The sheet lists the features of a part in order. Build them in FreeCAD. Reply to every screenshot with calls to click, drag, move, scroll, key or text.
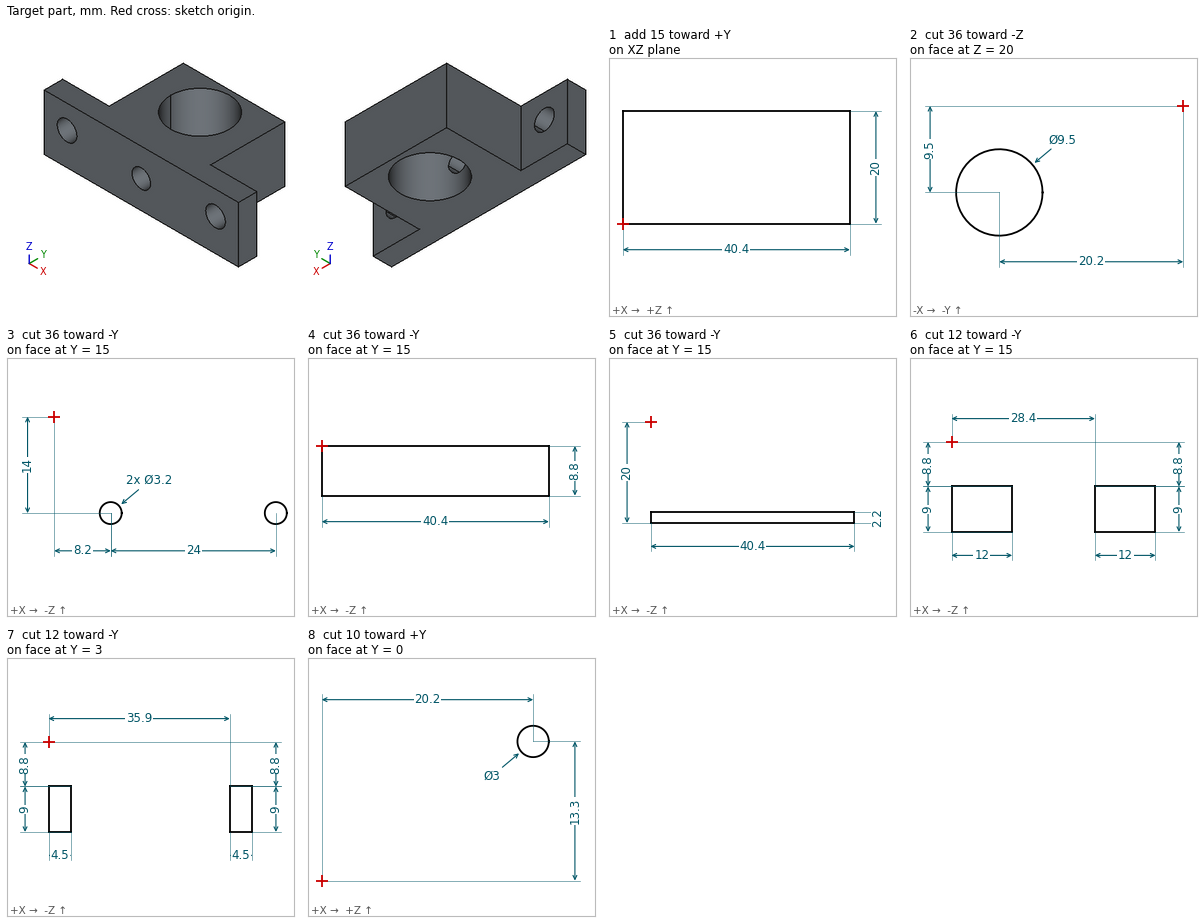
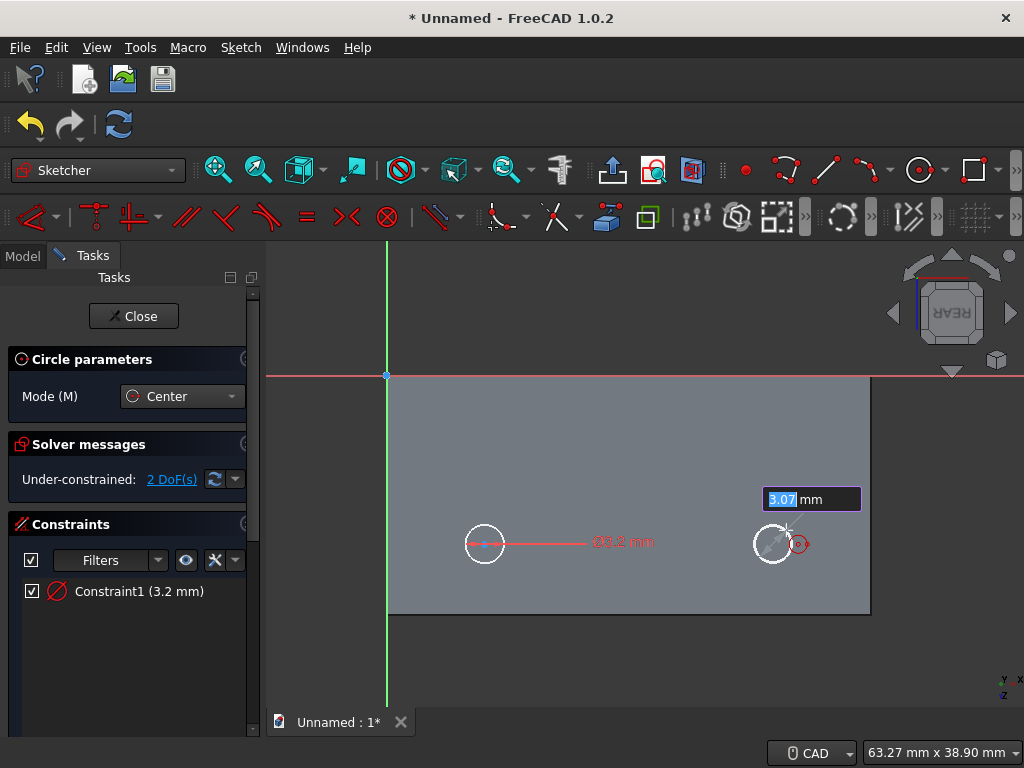
text(3.2)
key(Return)
key(Escape)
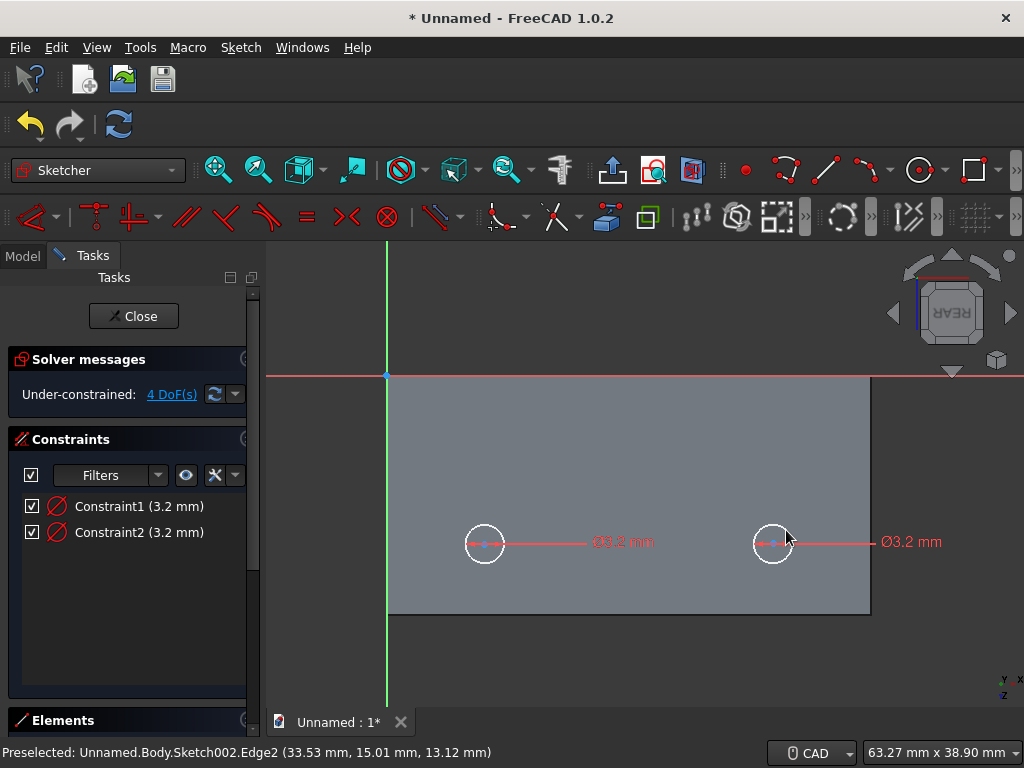
click(485, 544)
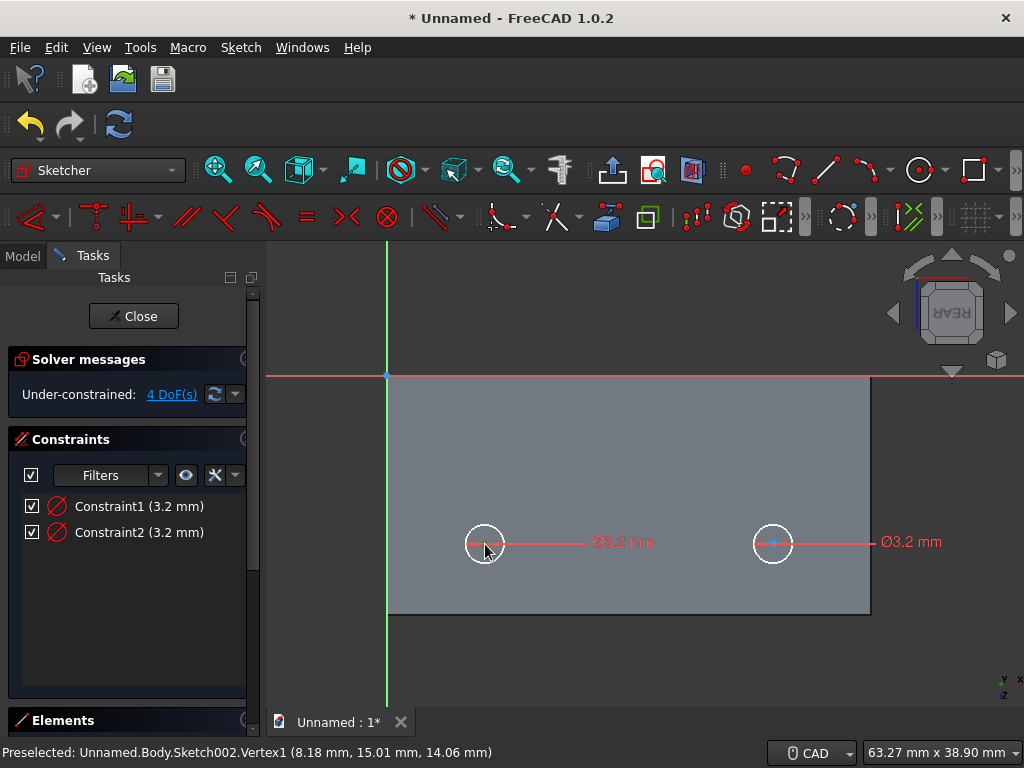
click(773, 544)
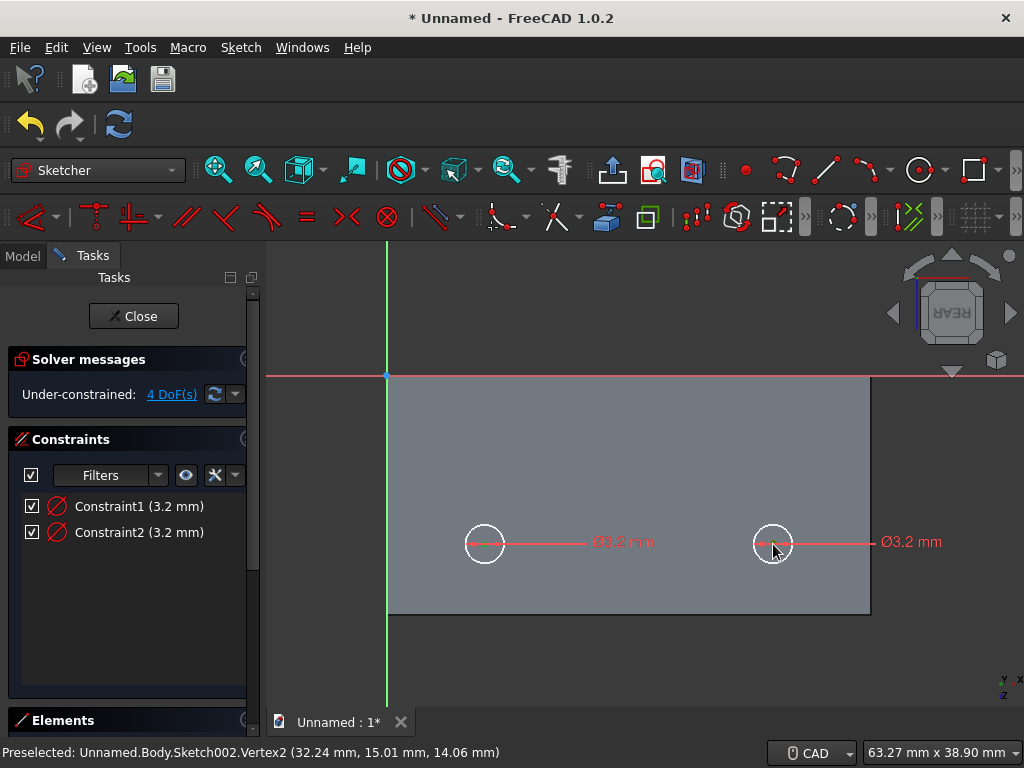
key(h)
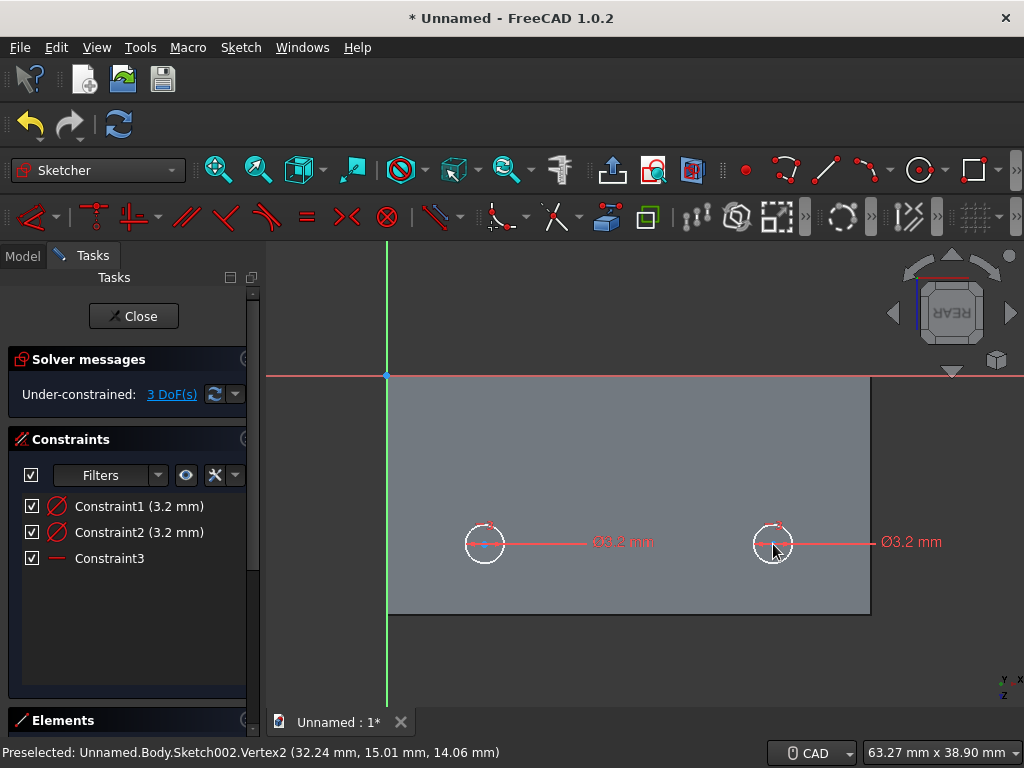
click(485, 544)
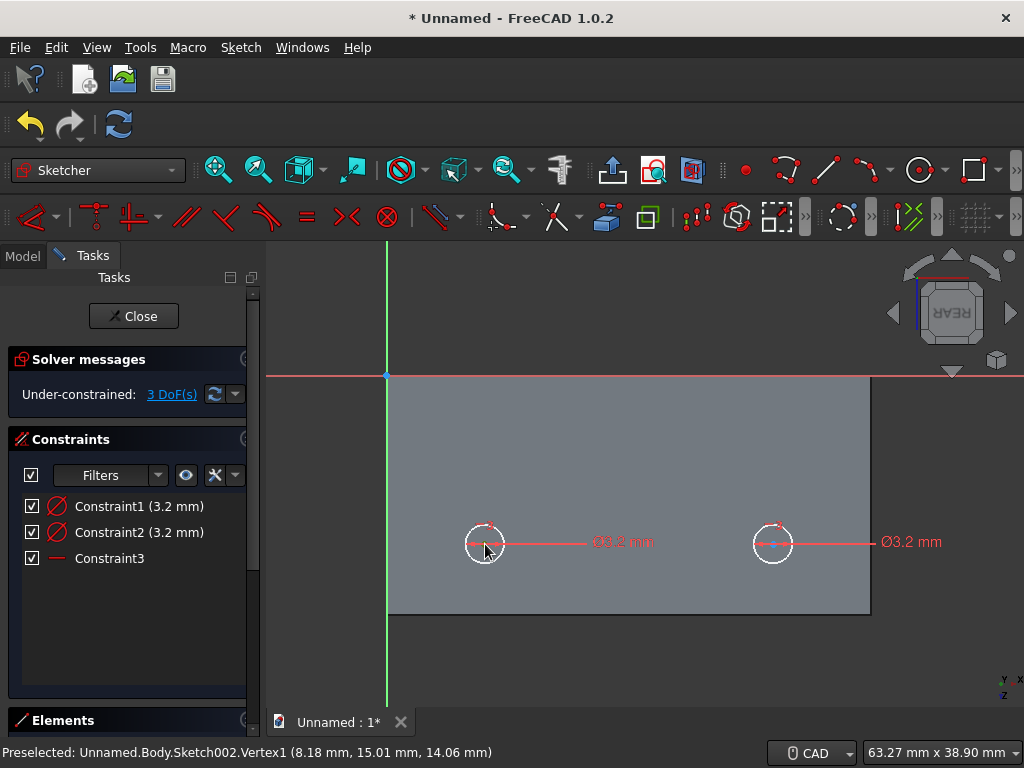
key(i)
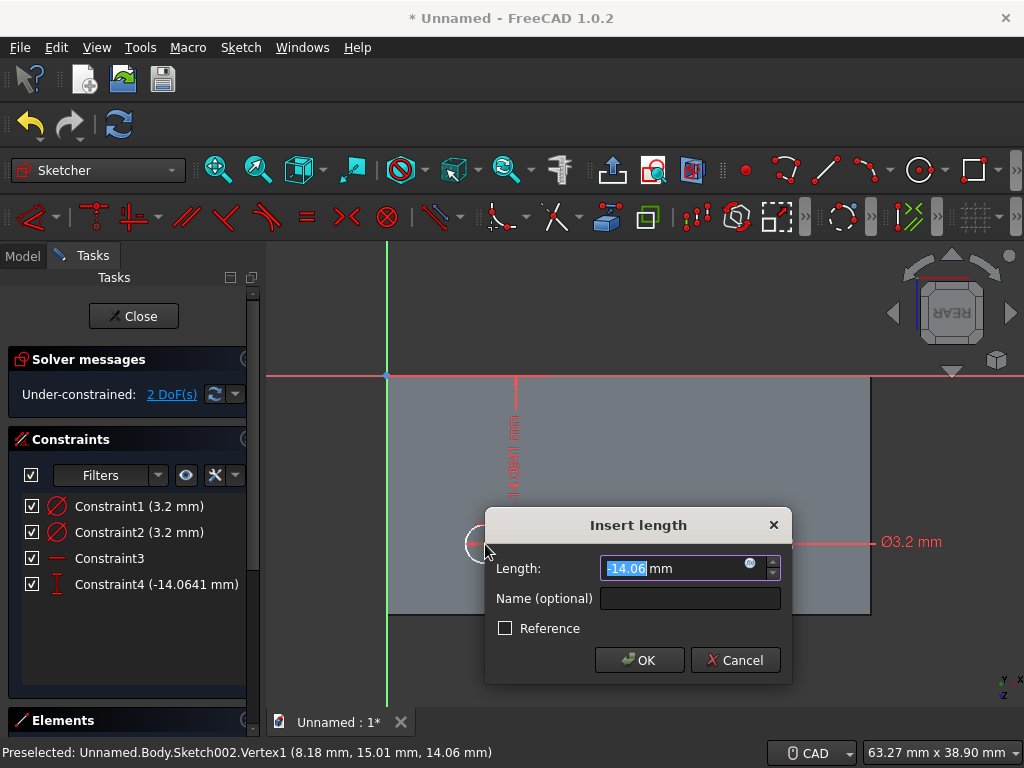
text(-14)
key(Return)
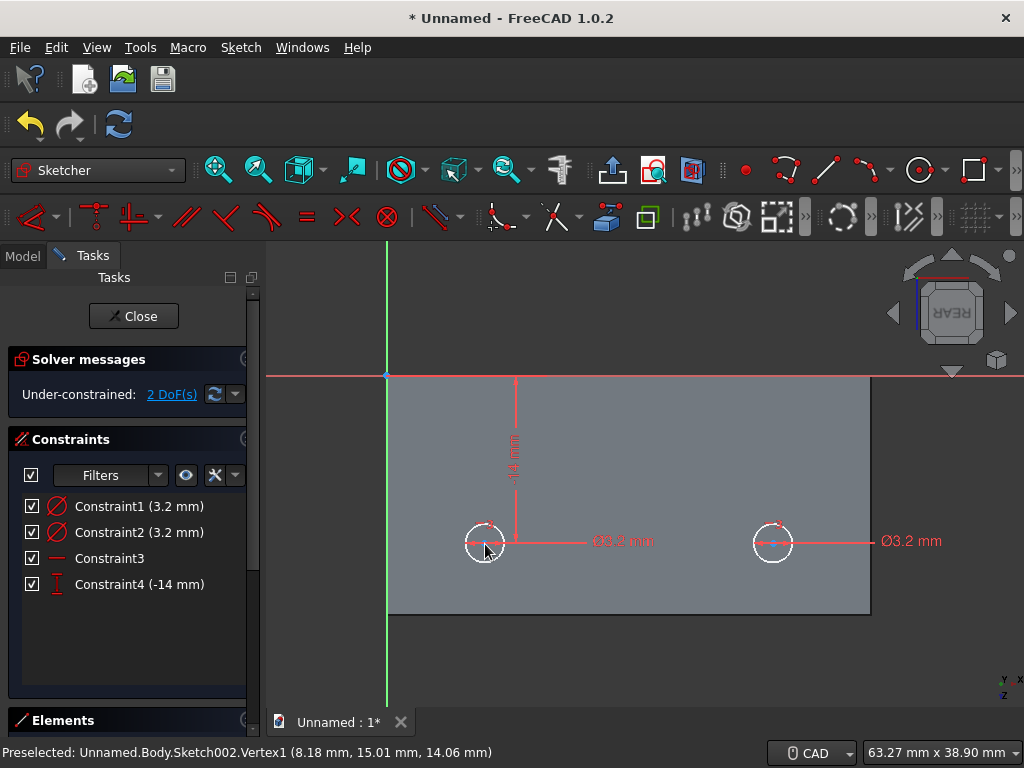
click(485, 543)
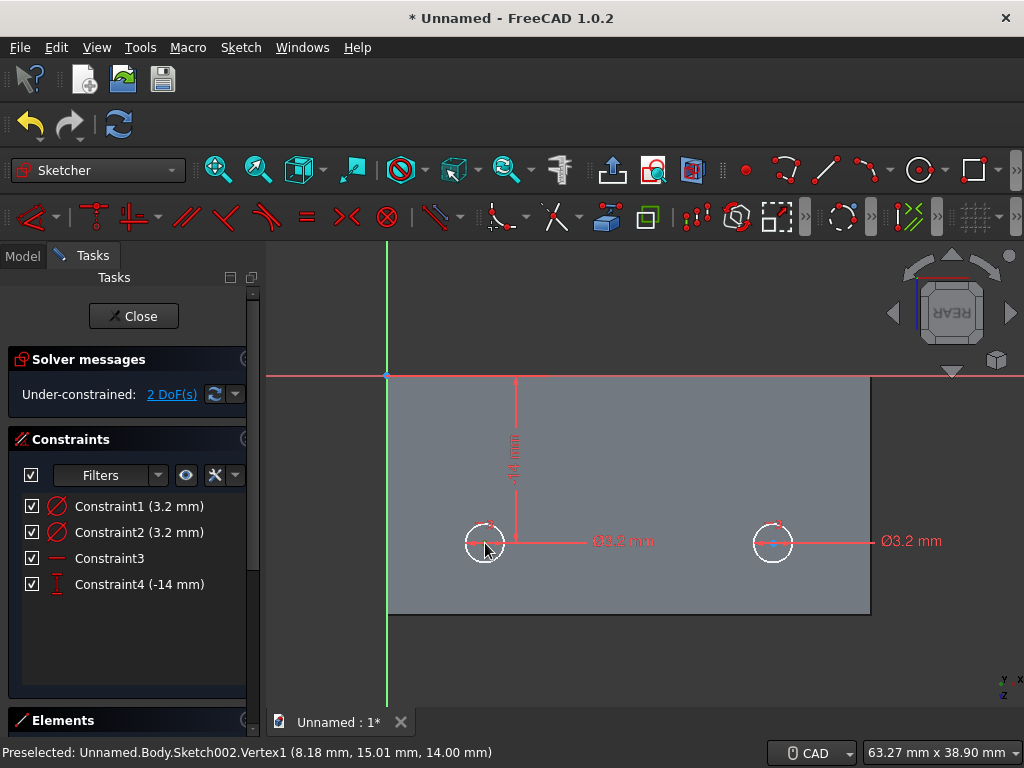
key(l)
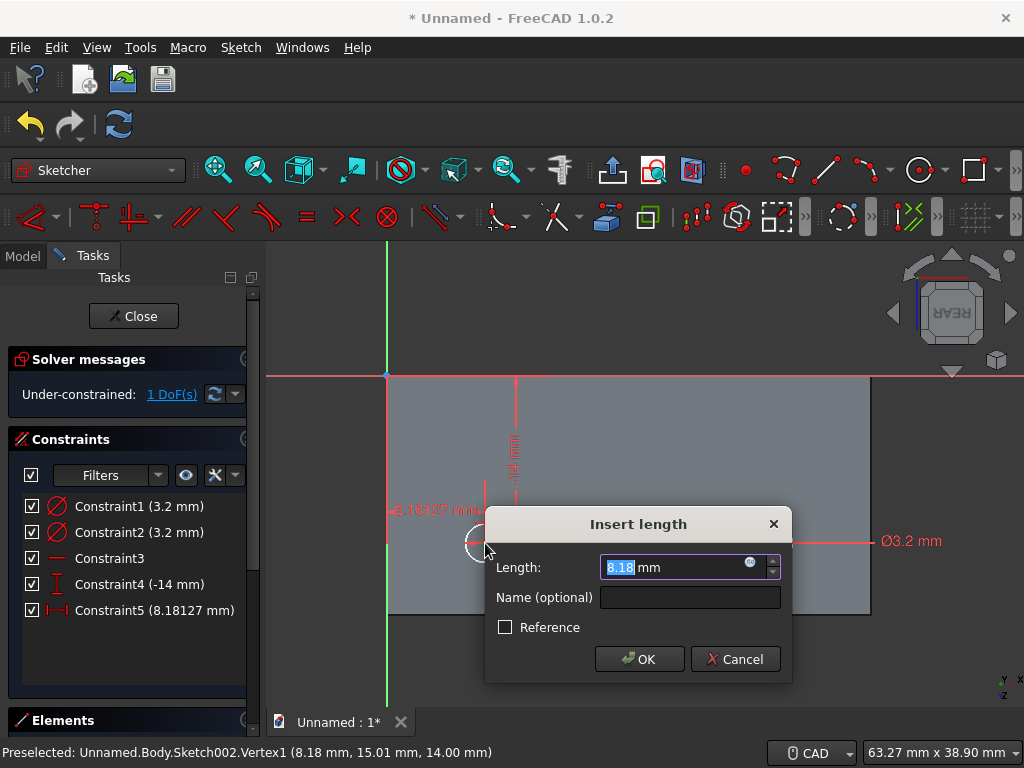
text(8.2)
key(Return)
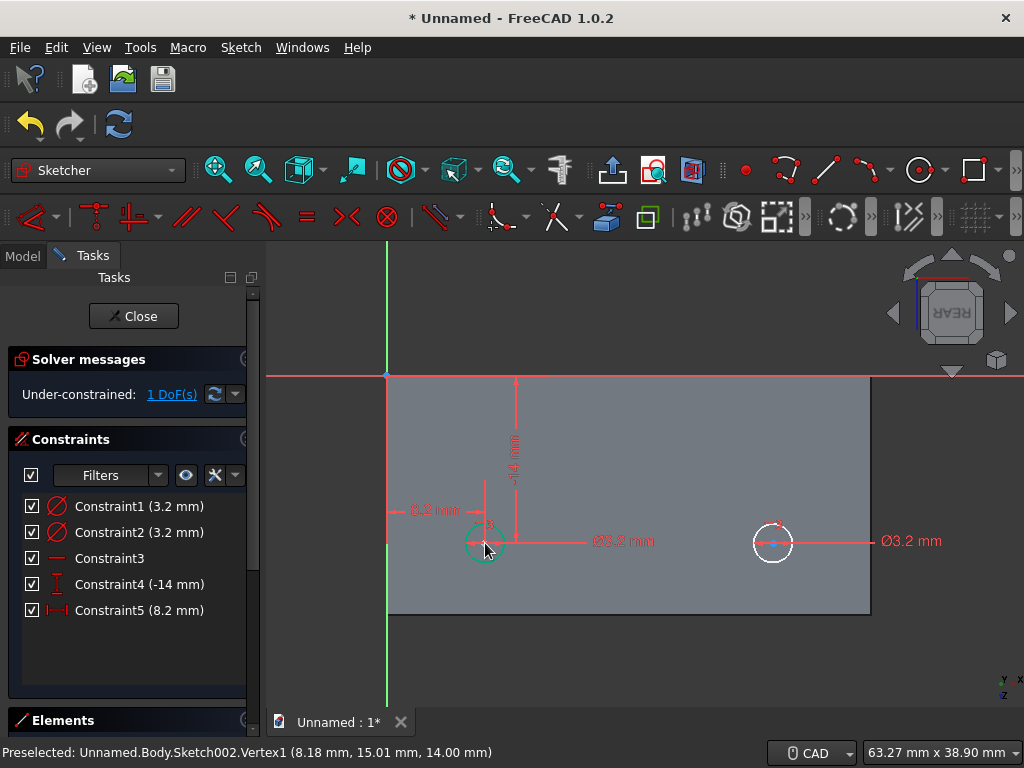
click(485, 543)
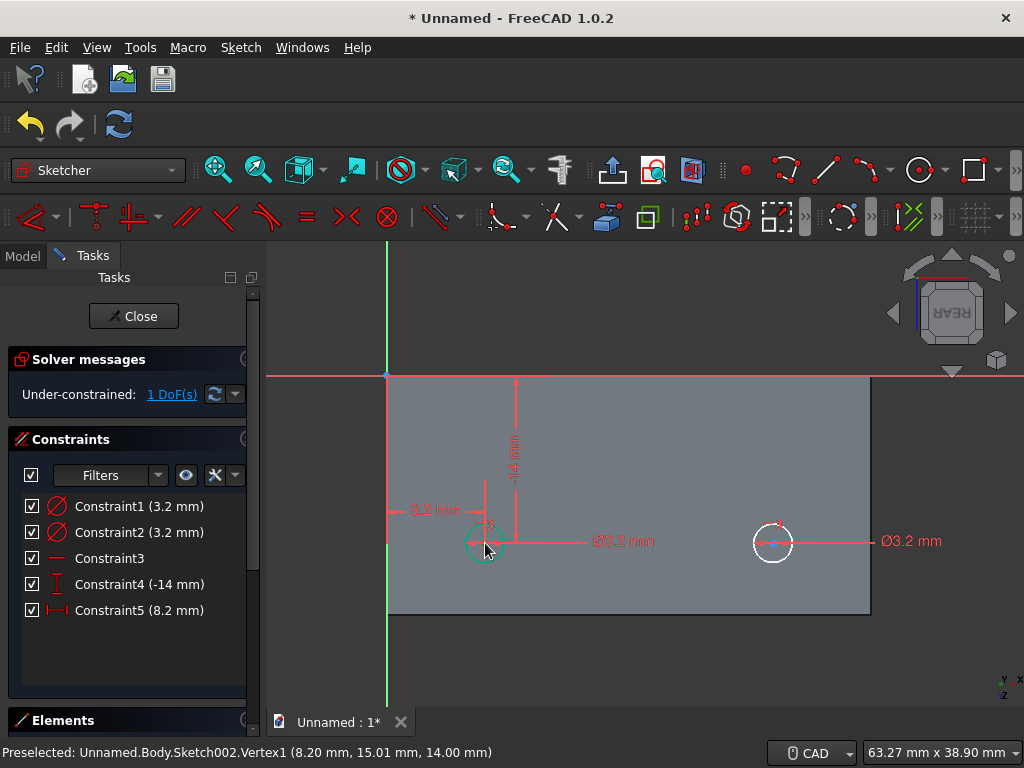
click(773, 543)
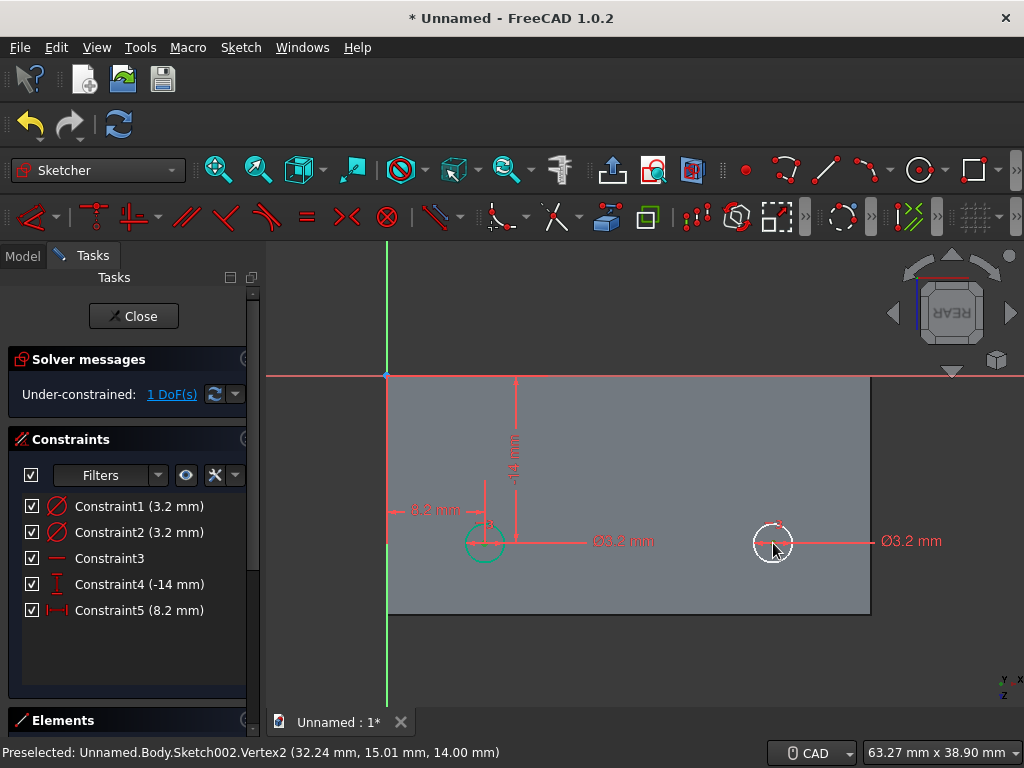
key(l)